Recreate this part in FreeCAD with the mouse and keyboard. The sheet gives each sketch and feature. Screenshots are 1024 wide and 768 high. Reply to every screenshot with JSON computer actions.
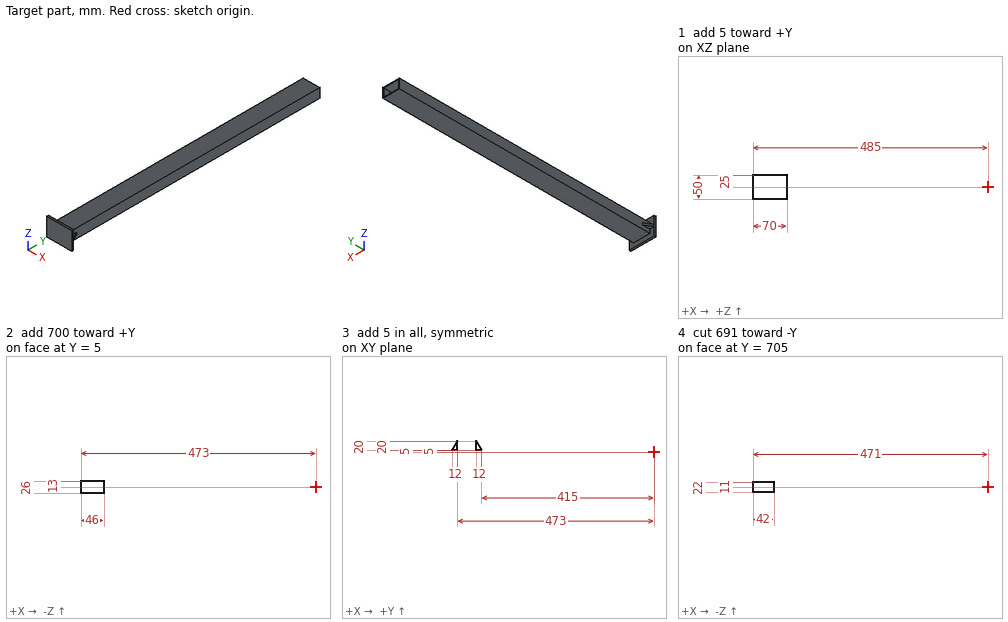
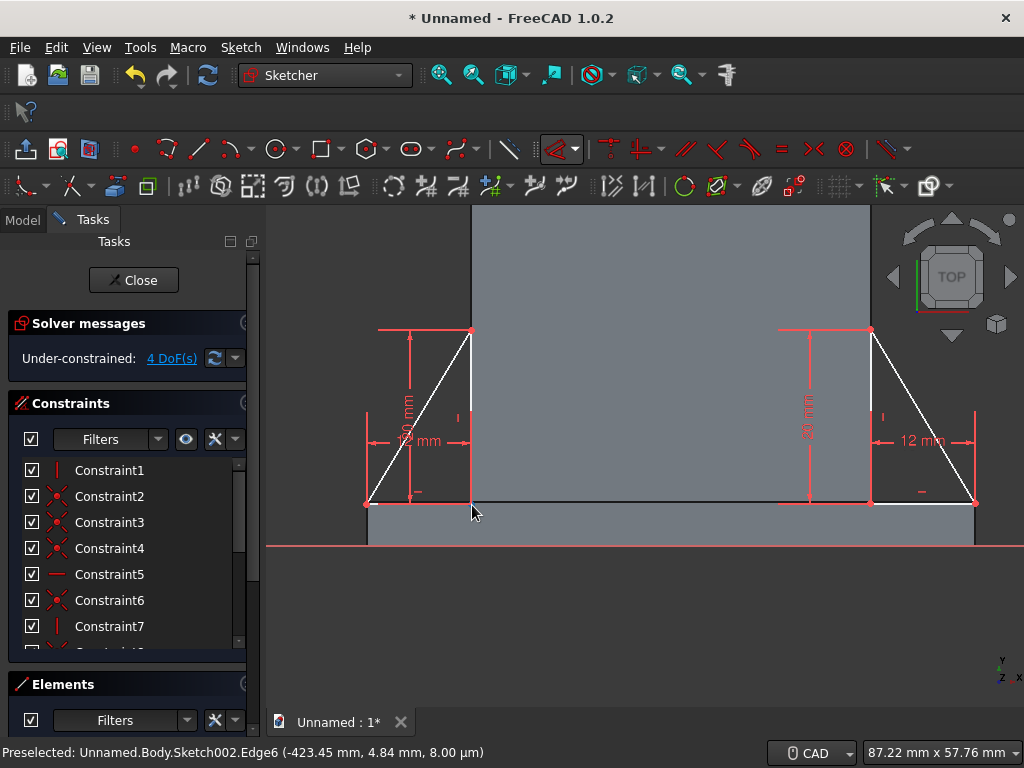
{"action": "left_click", "coordinate": [471, 504]}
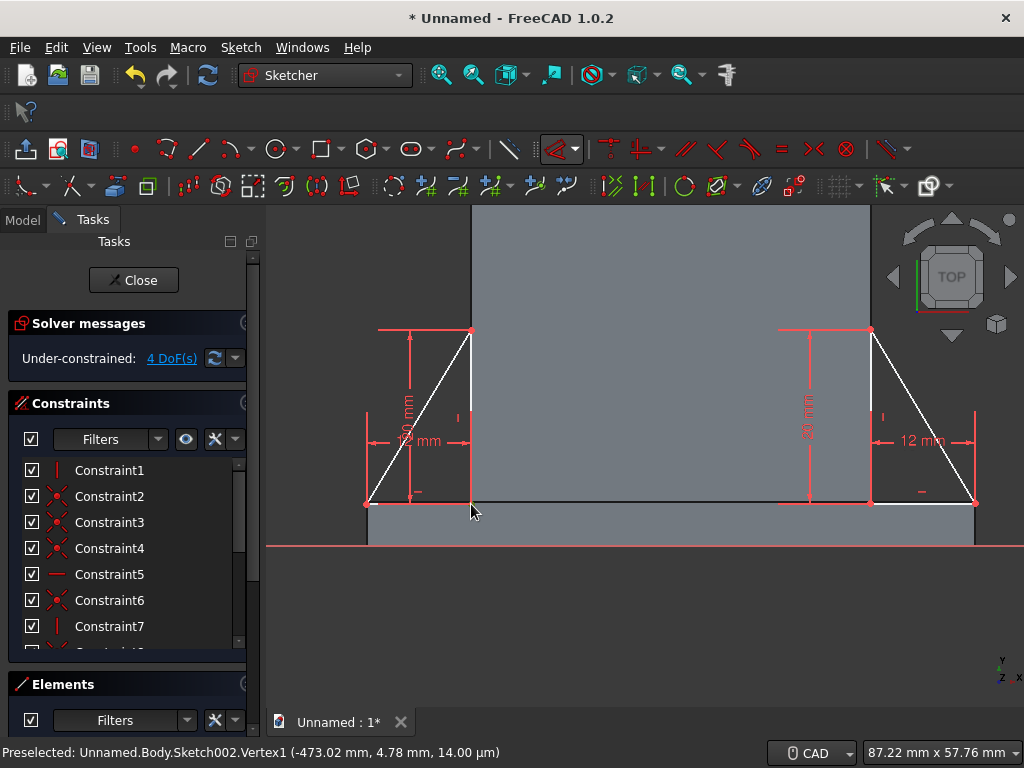
{"action": "key", "text": "i"}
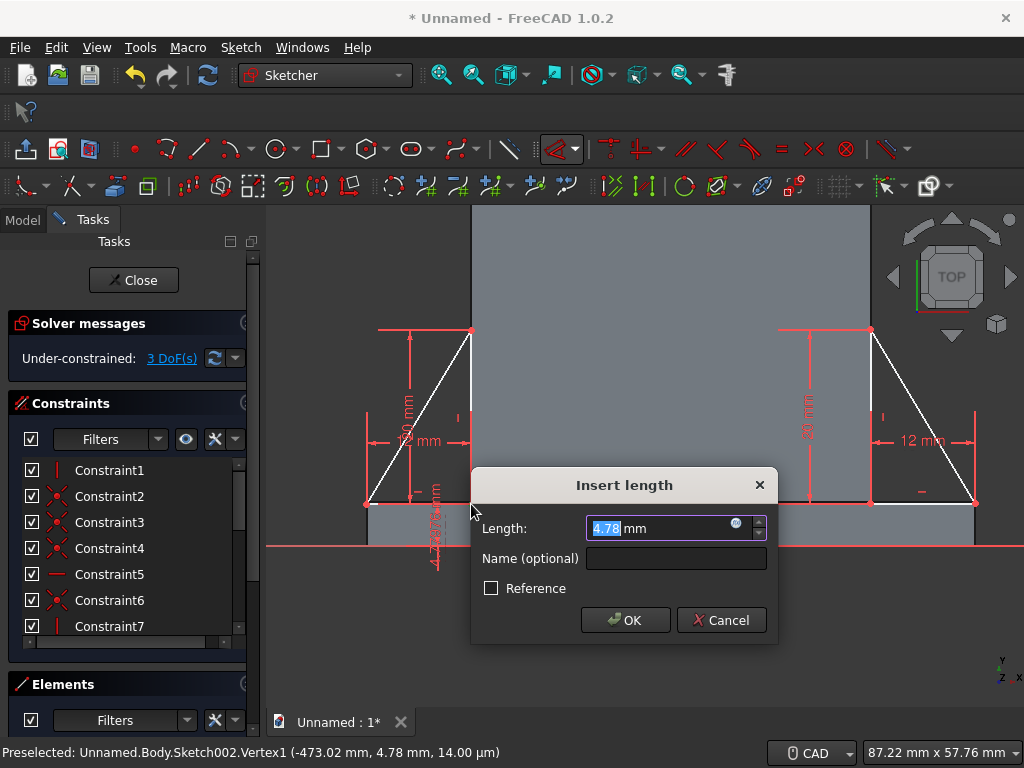
{"action": "type", "text": "5"}
{"action": "key", "text": "Return"}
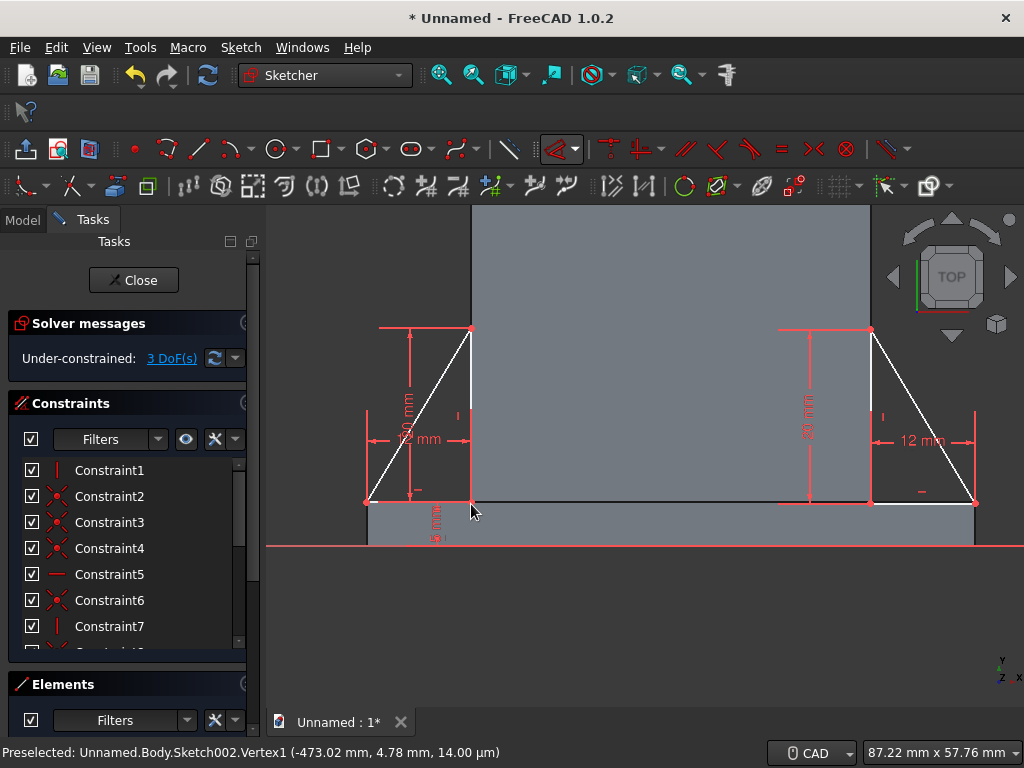
{"action": "scroll", "coordinate": [384, 539], "scroll_direction": "down", "scroll_amount": 2}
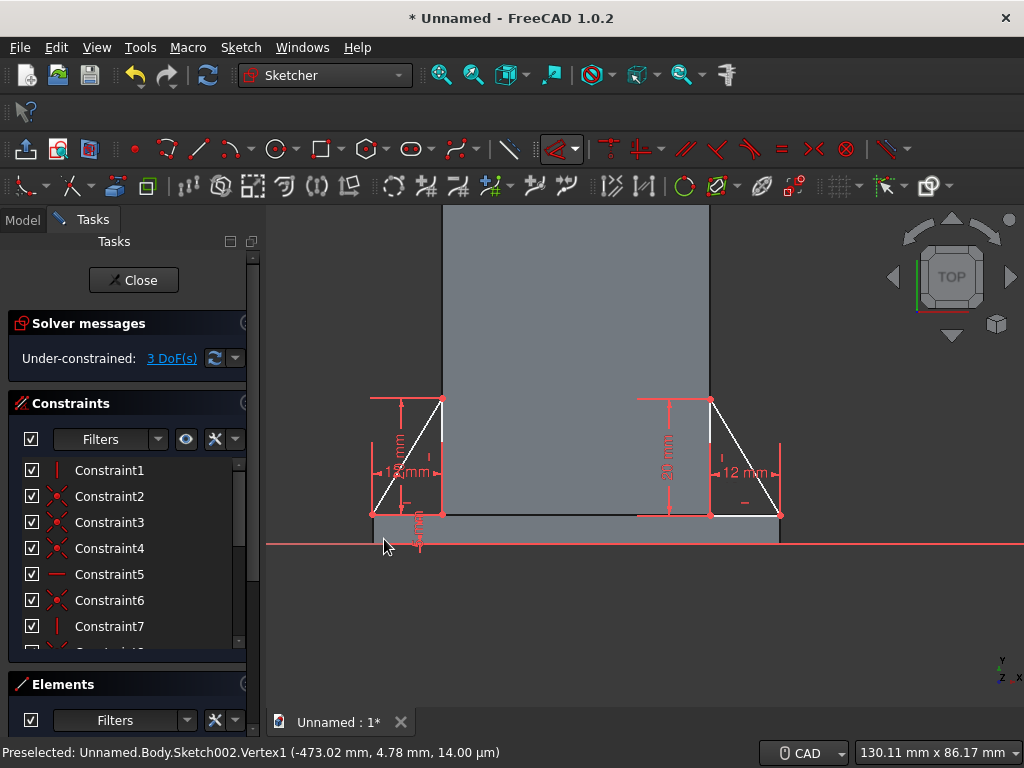
{"action": "scroll", "coordinate": [780, 516], "scroll_direction": "up", "scroll_amount": 2}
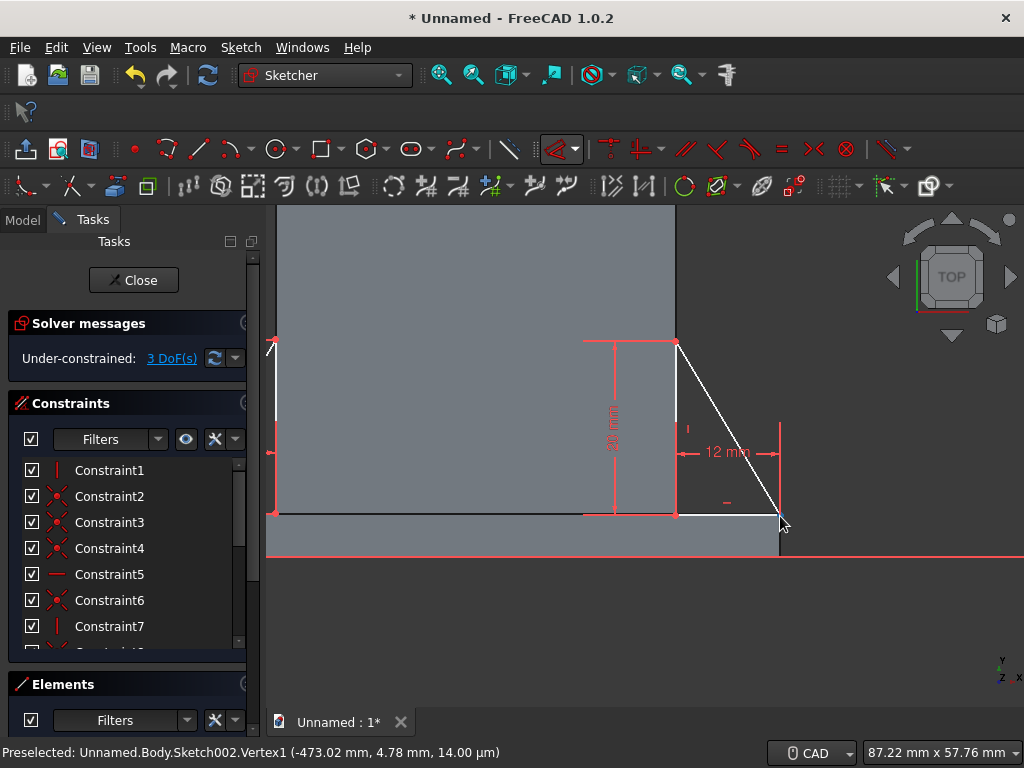
{"action": "left_click", "coordinate": [780, 515]}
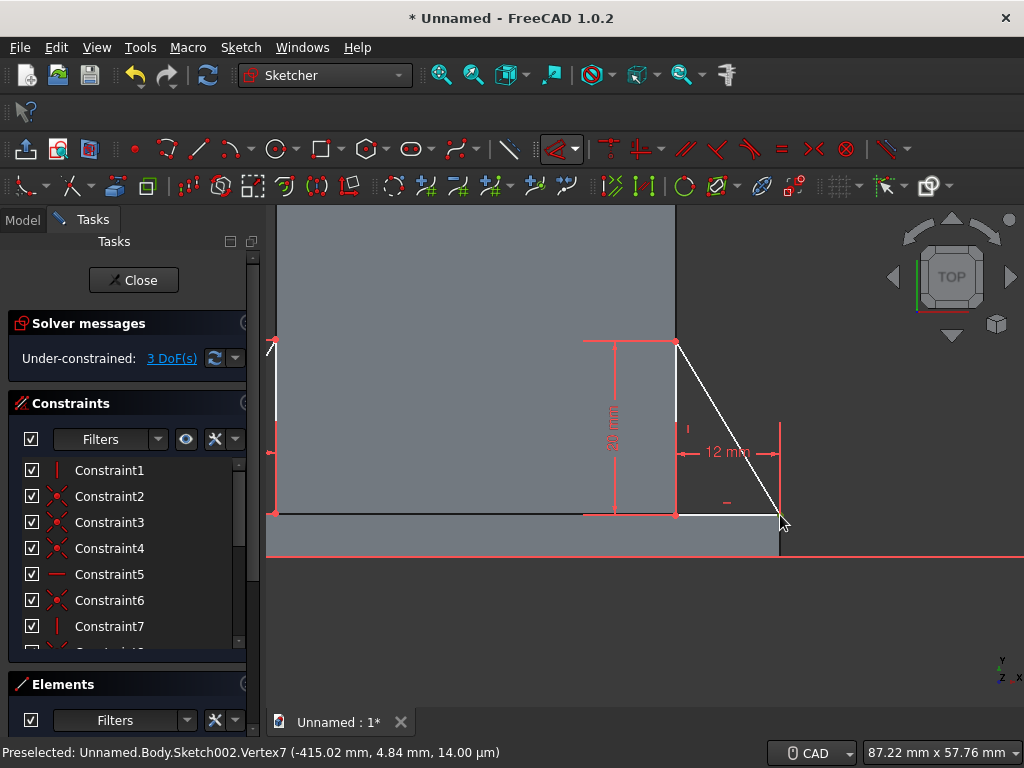
{"action": "left_click", "coordinate": [578, 150]}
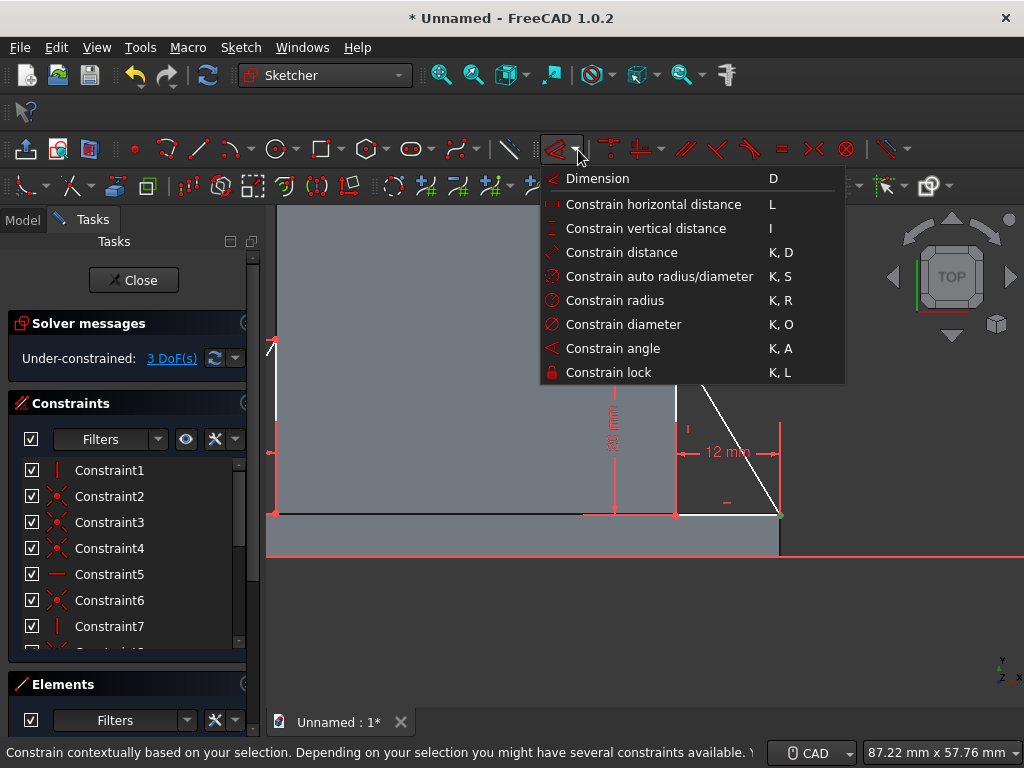
{"action": "left_click", "coordinate": [693, 228]}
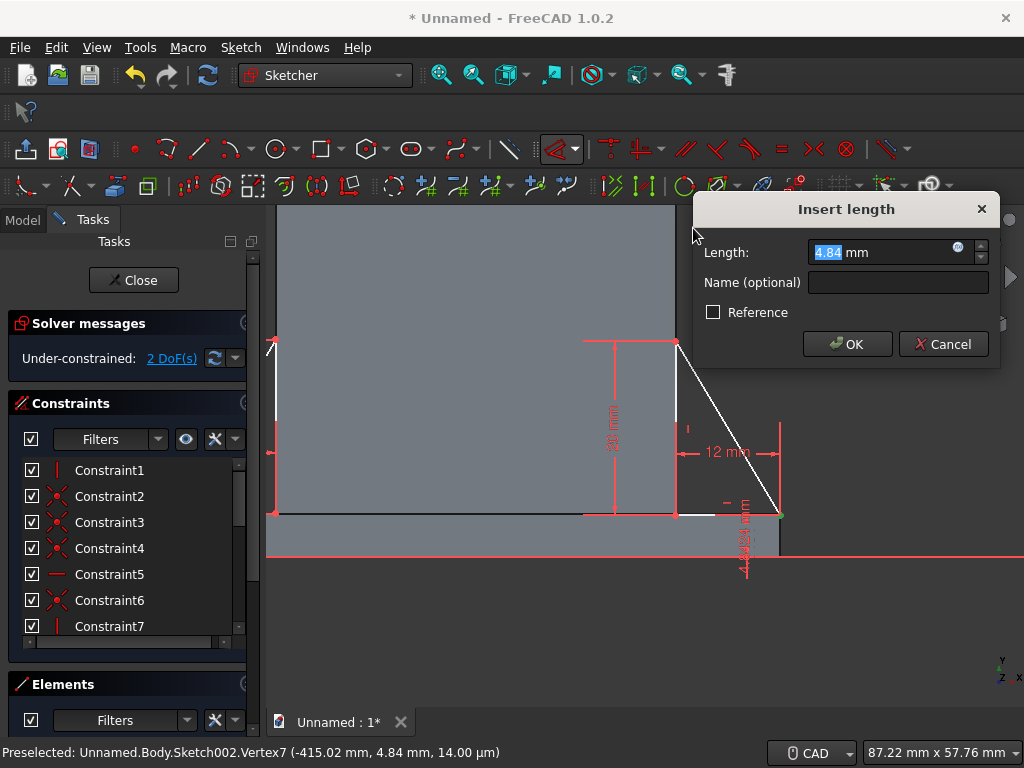
{"action": "type", "text": "5"}
{"action": "key", "text": "Return"}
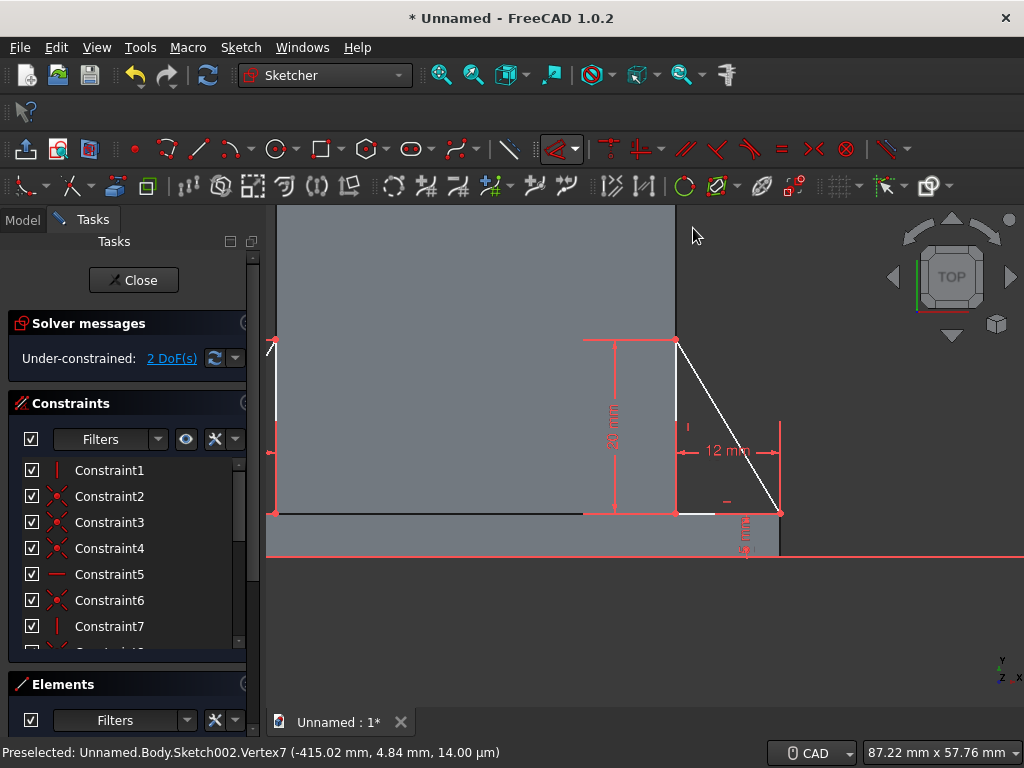
{"action": "scroll", "coordinate": [781, 515], "scroll_direction": "down", "scroll_amount": 2}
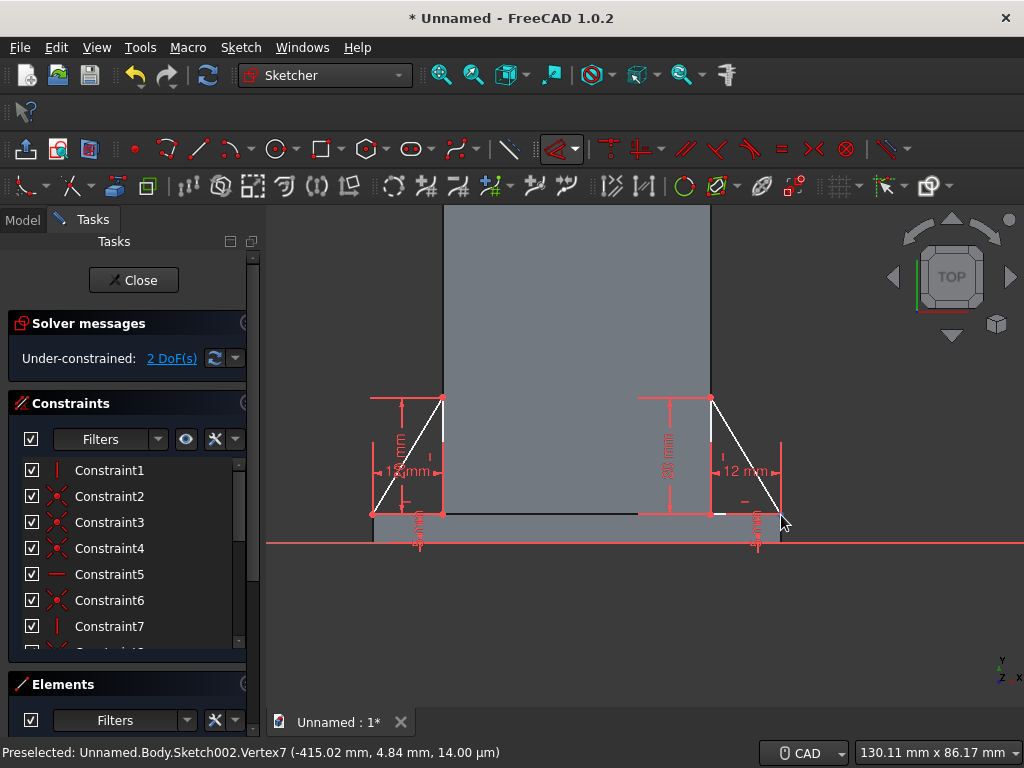
{"action": "left_click", "coordinate": [443, 514]}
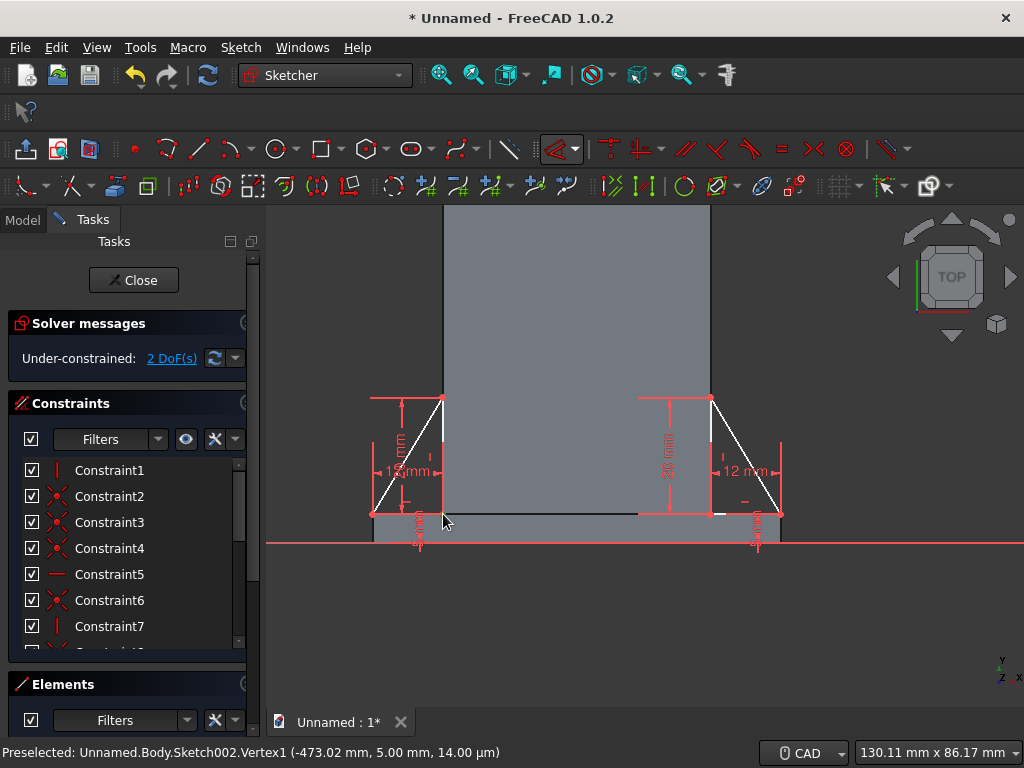
{"action": "key", "text": "l"}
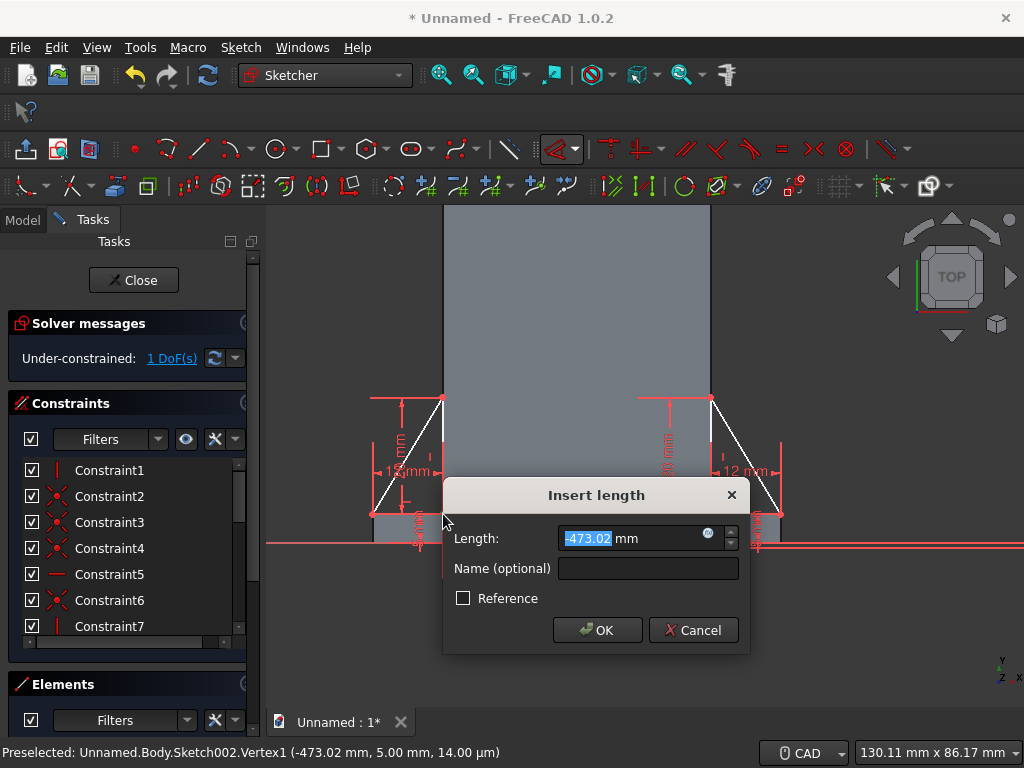
{"action": "type", "text": "-473"}
{"action": "key", "text": "Return"}